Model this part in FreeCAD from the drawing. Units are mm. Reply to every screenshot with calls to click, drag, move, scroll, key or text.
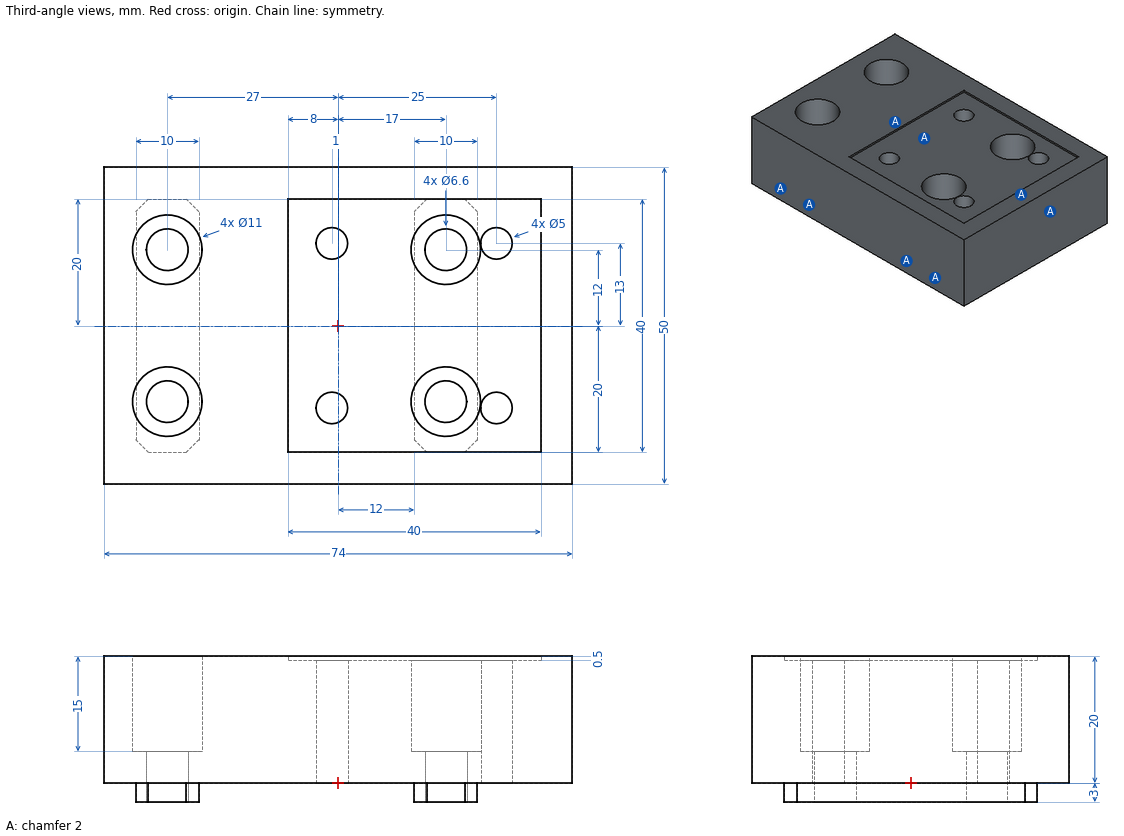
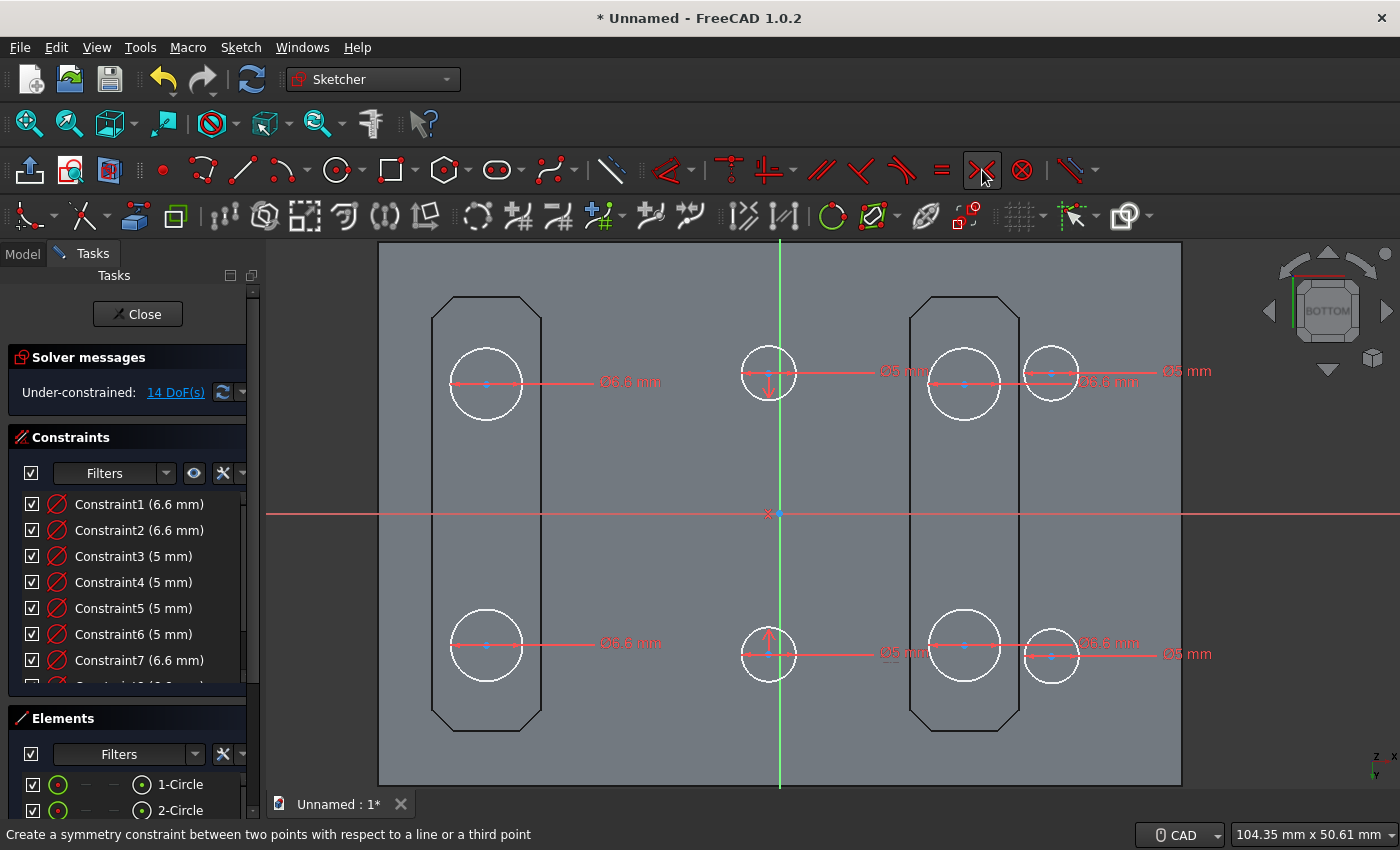
click(1052, 656)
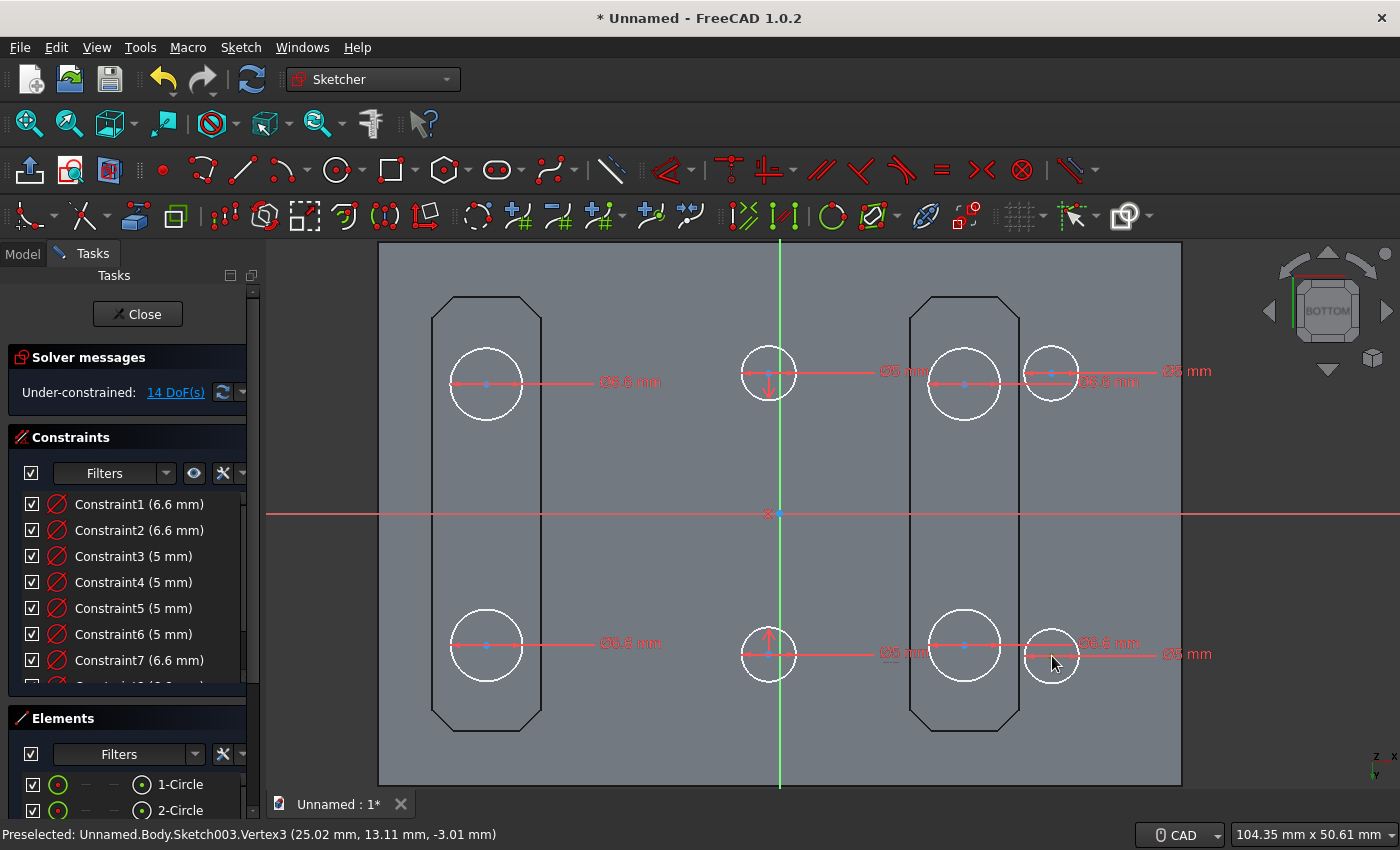
click(1051, 373)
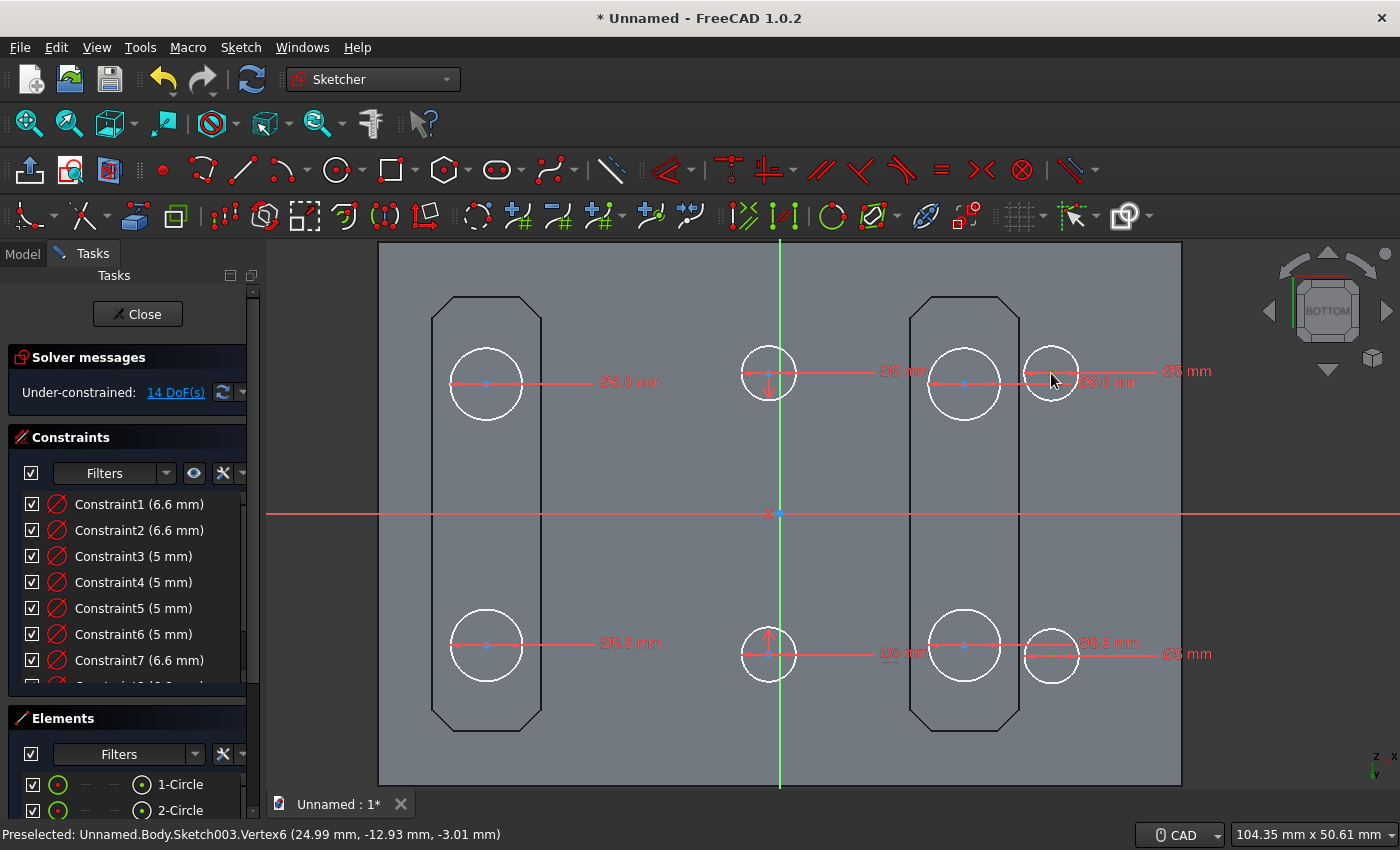
click(361, 514)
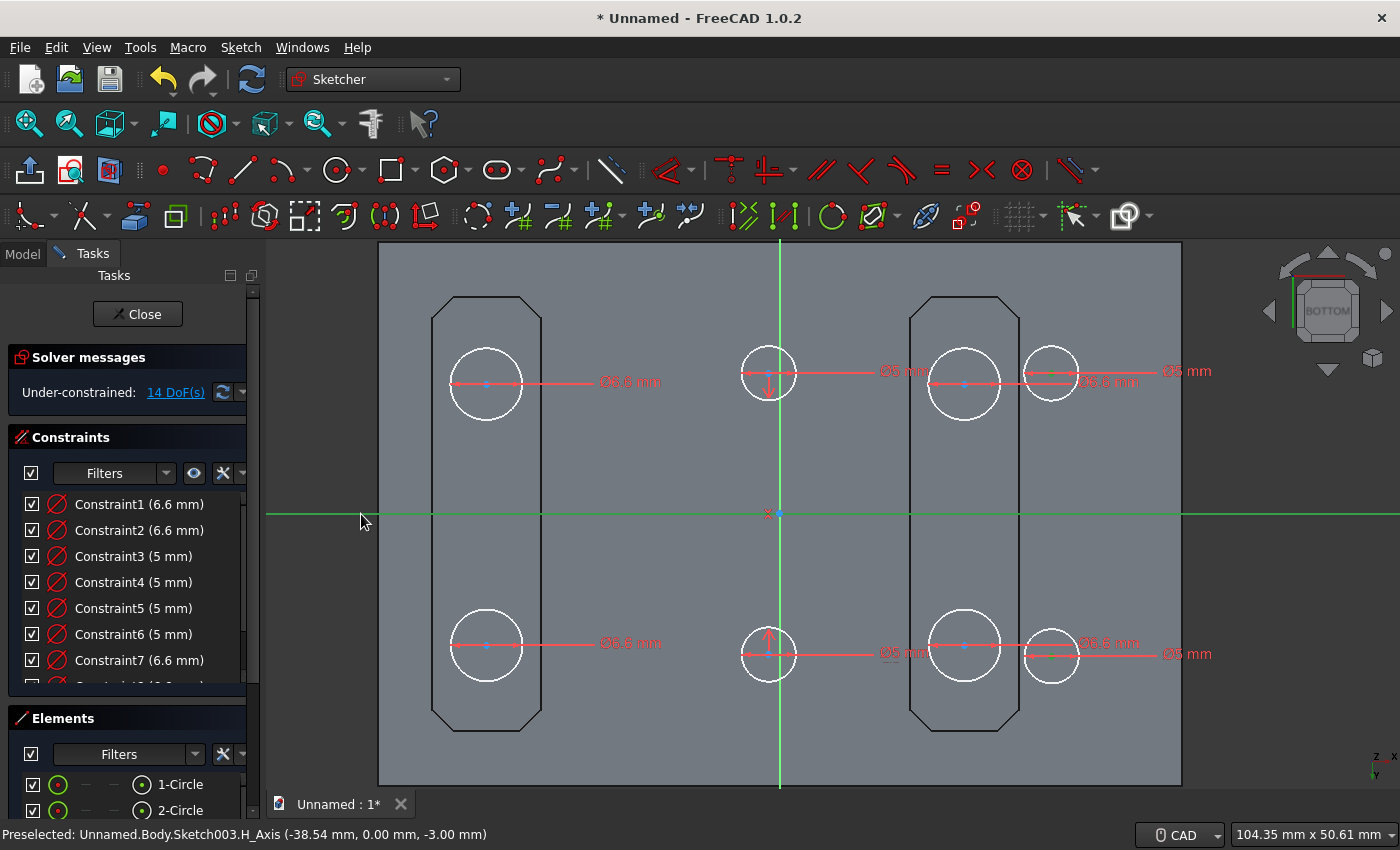
click(982, 170)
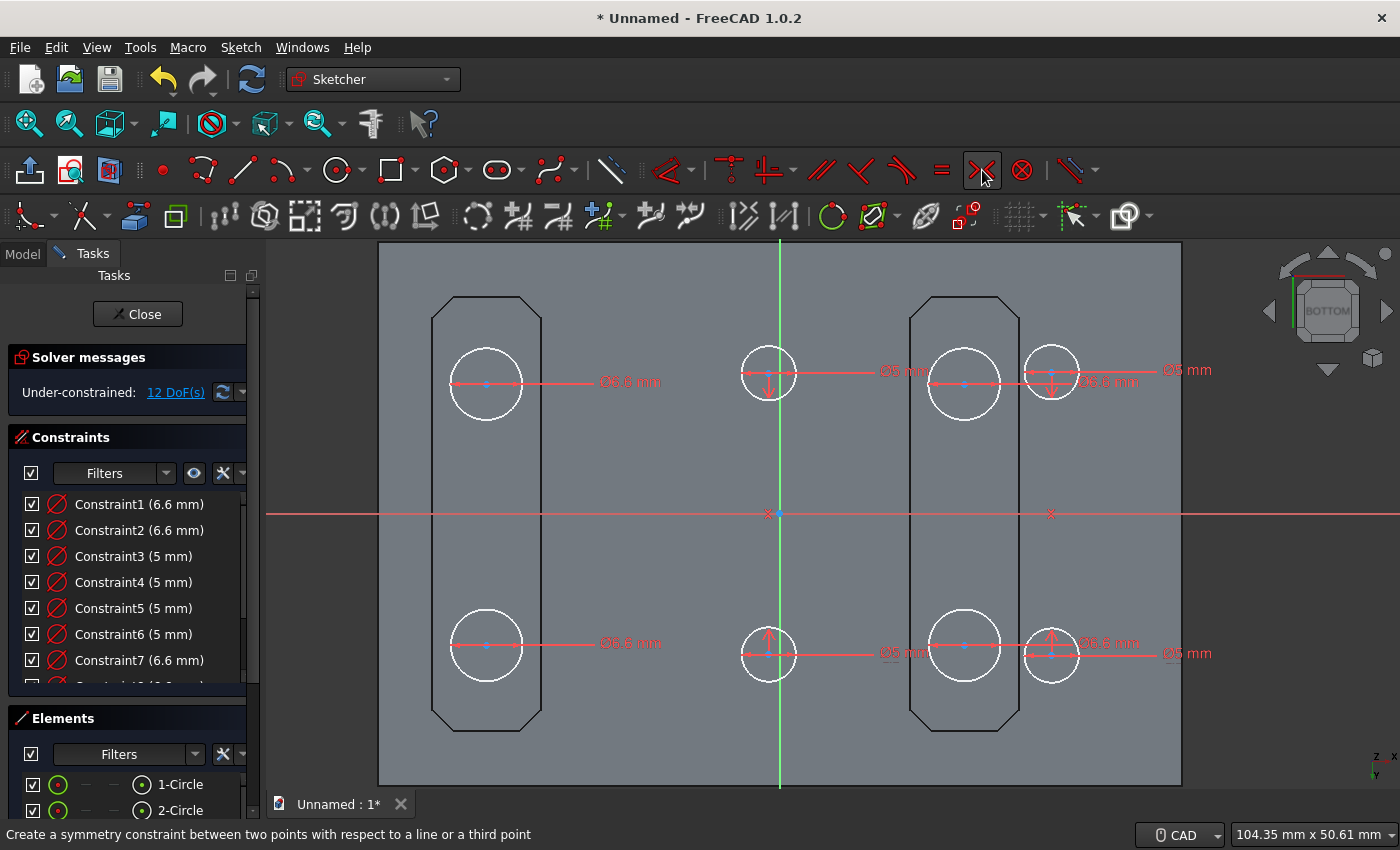
click(487, 645)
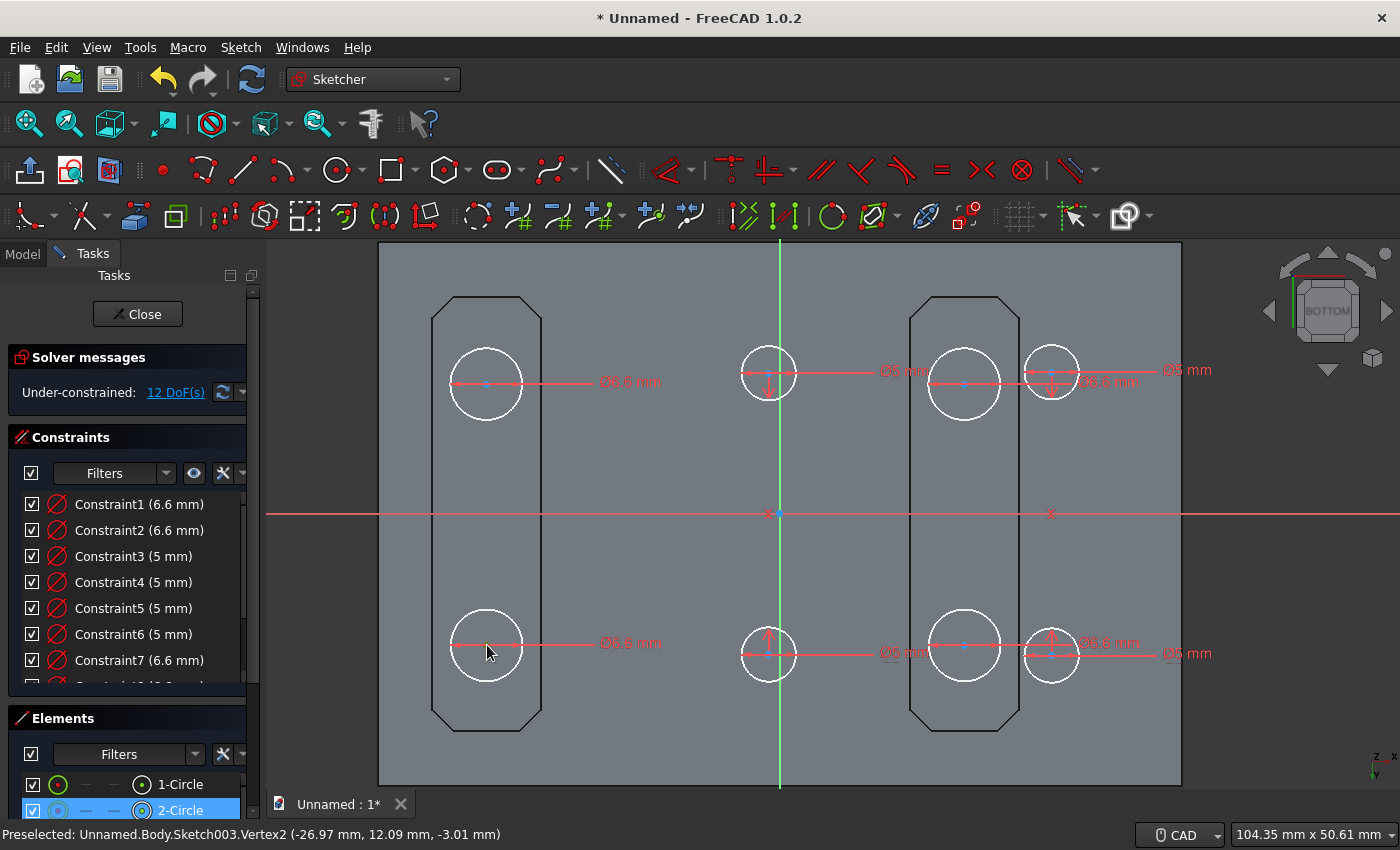
click(486, 384)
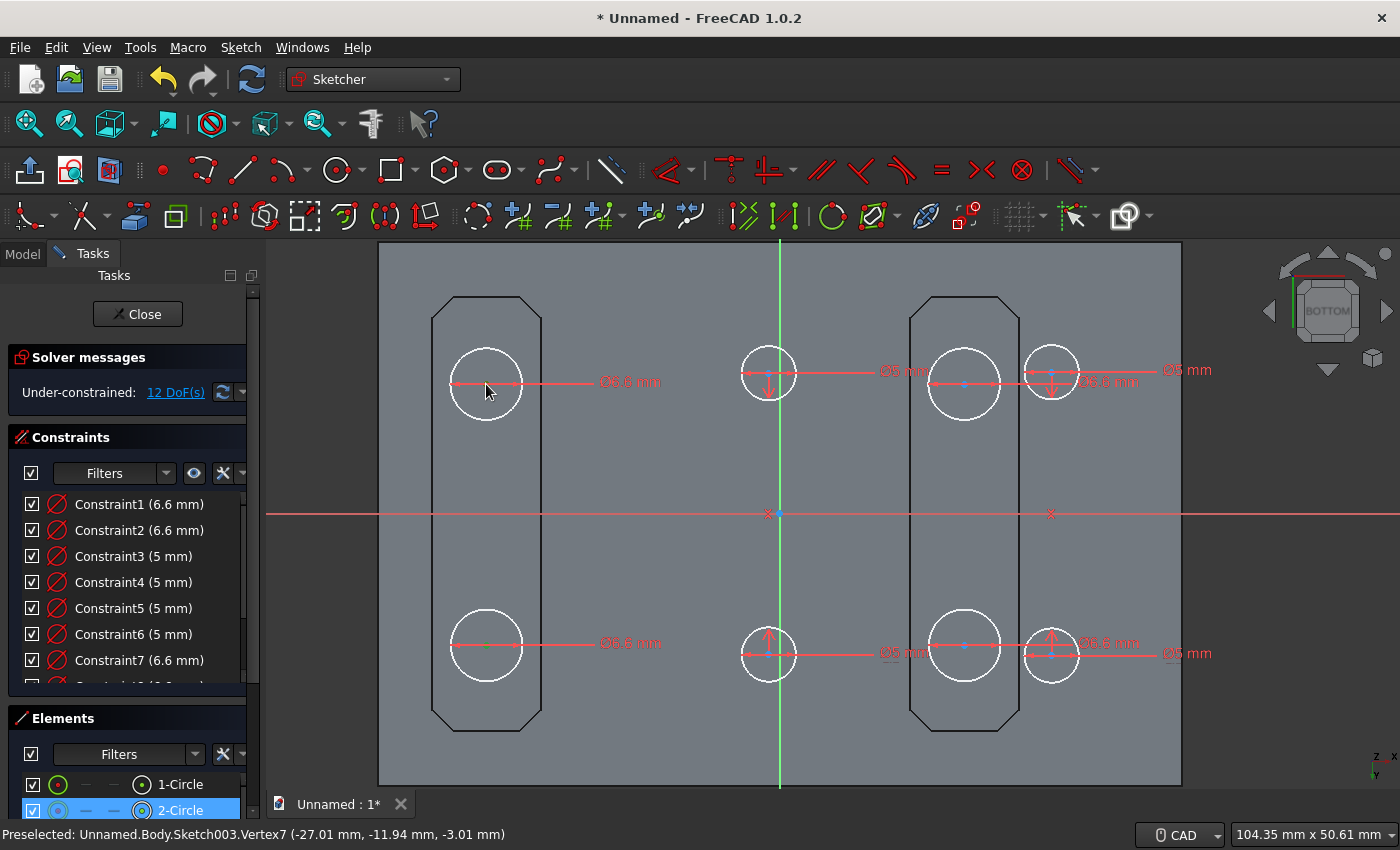
click(361, 514)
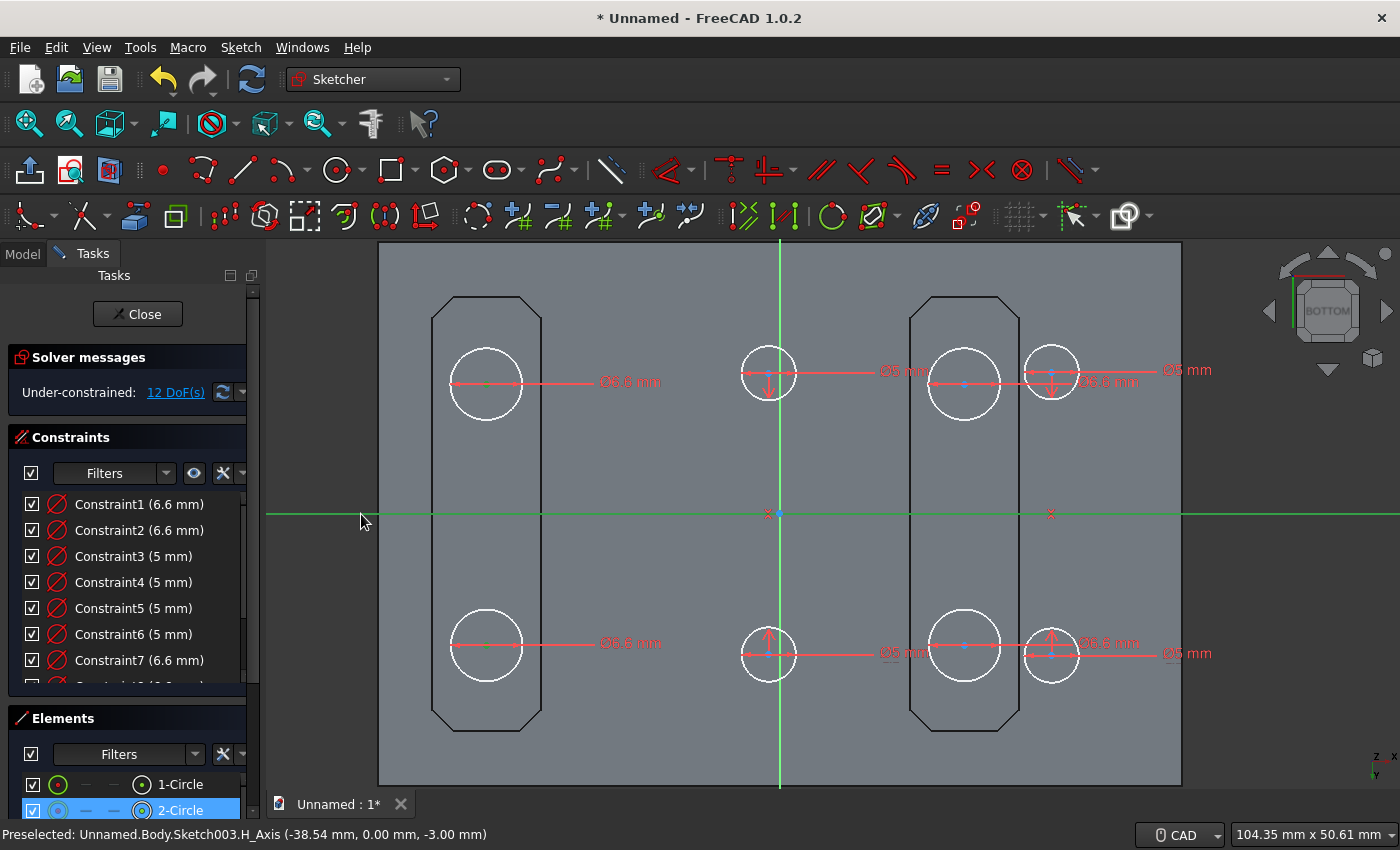
click(982, 170)